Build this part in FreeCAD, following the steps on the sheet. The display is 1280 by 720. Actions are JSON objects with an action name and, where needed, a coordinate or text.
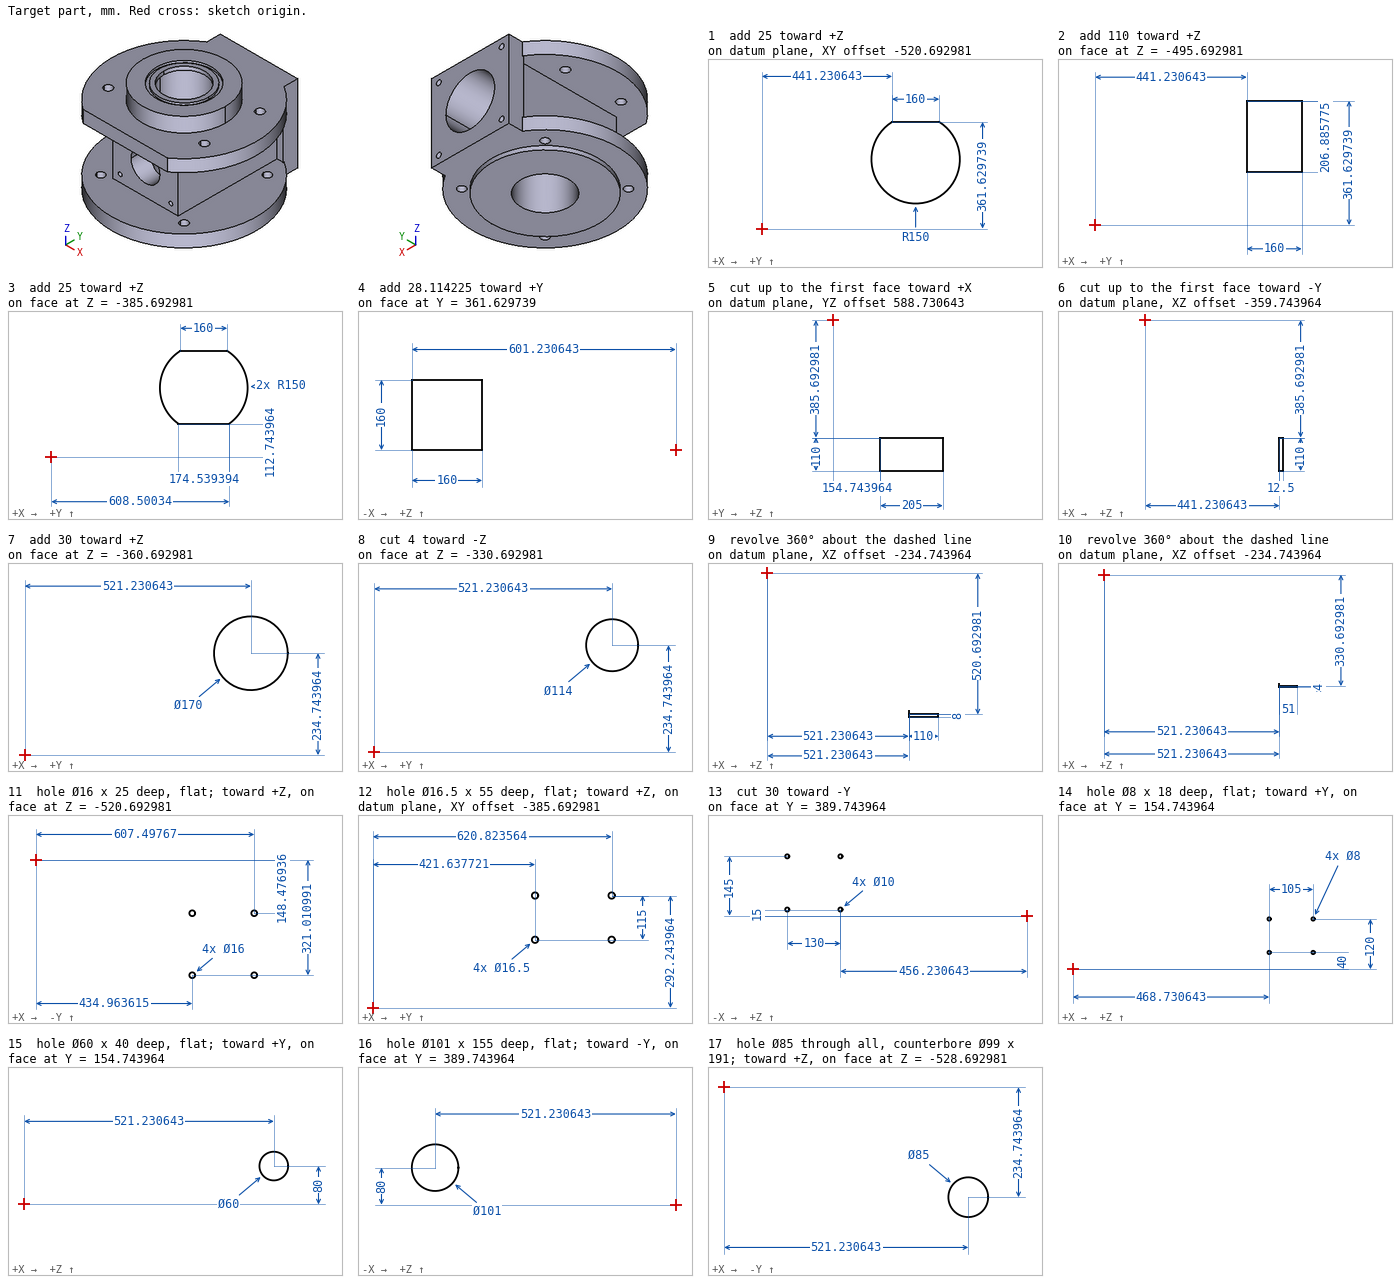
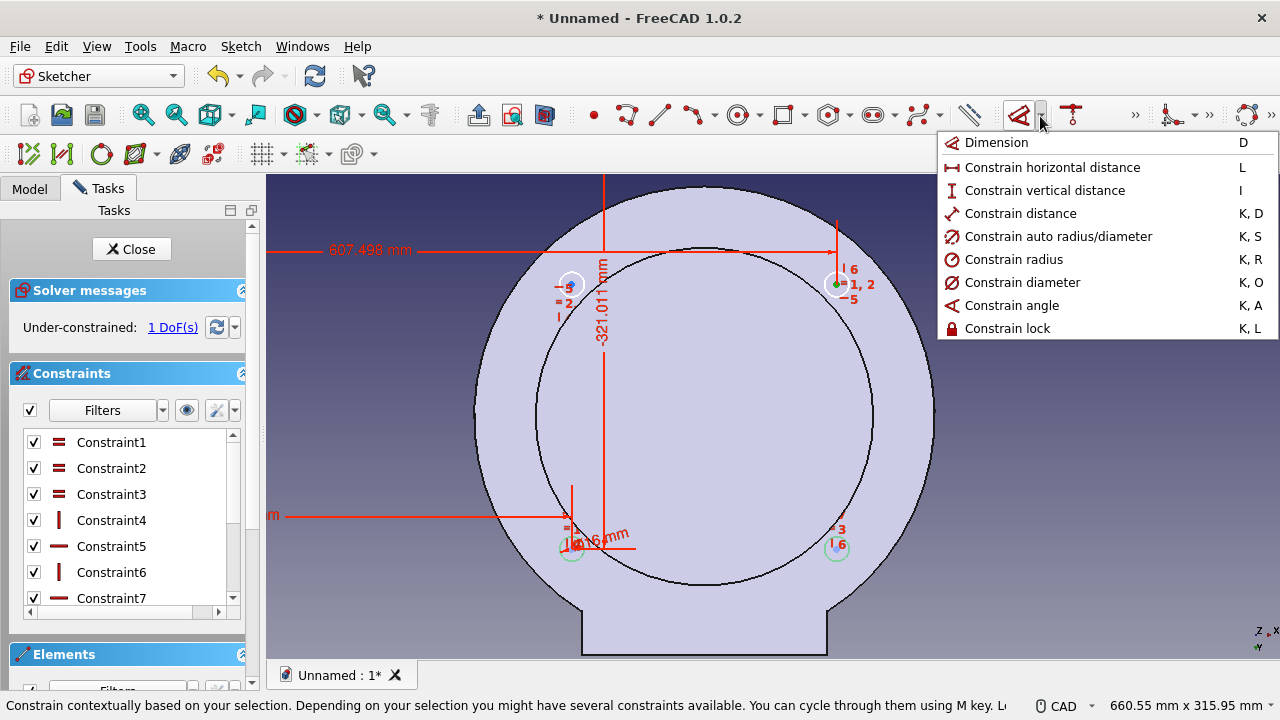
{"action": "left_click", "coordinate": [1108, 190]}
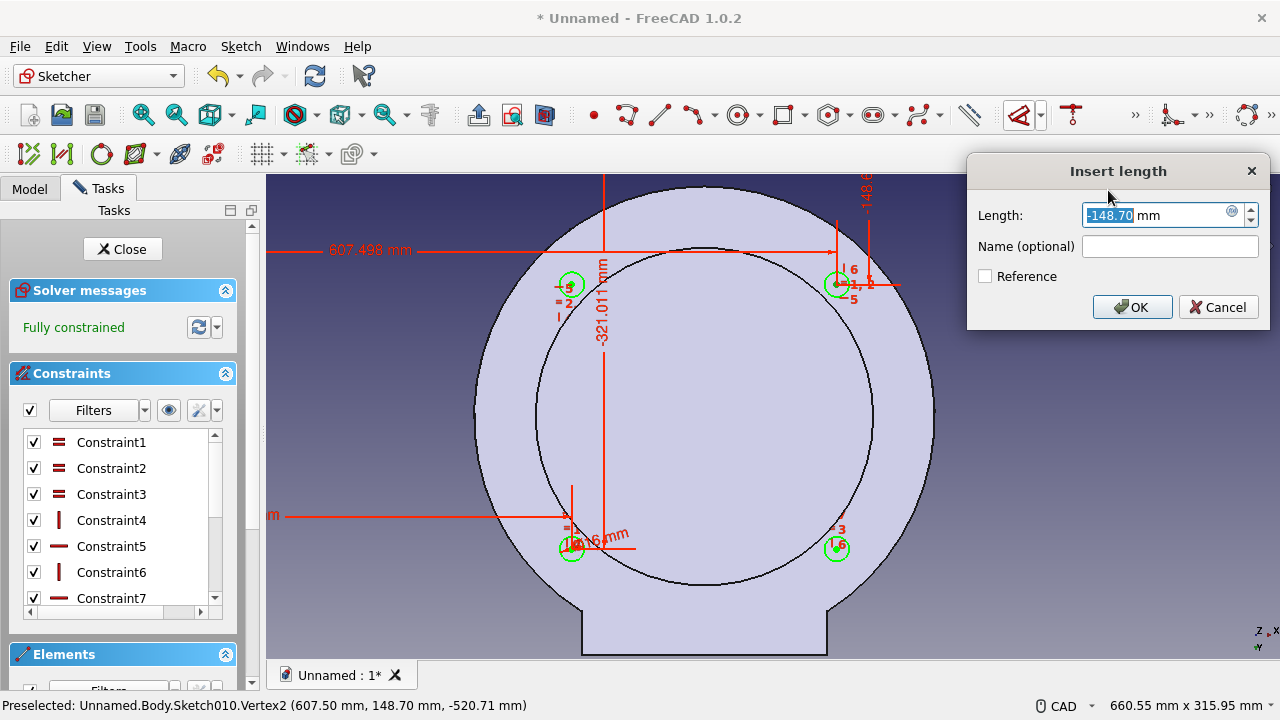
{"action": "type", "text": "-148.476936"}
{"action": "key", "text": "Return"}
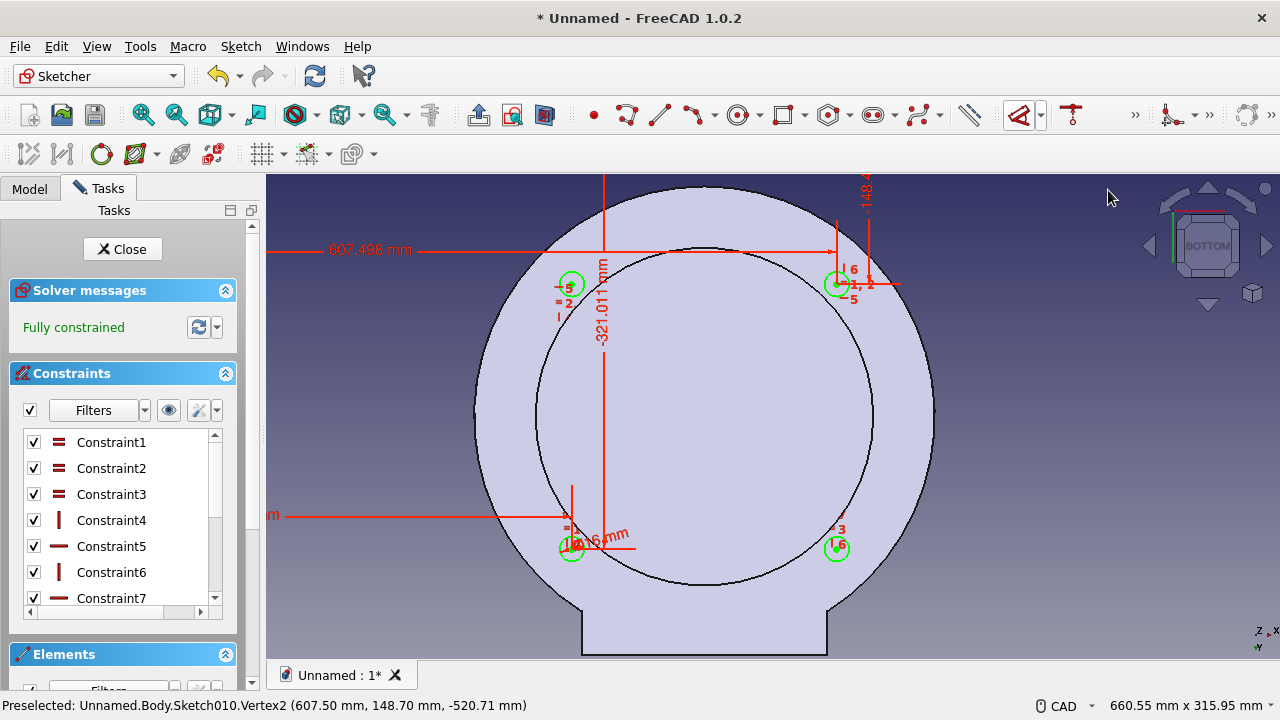
{"action": "left_click", "coordinate": [123, 249]}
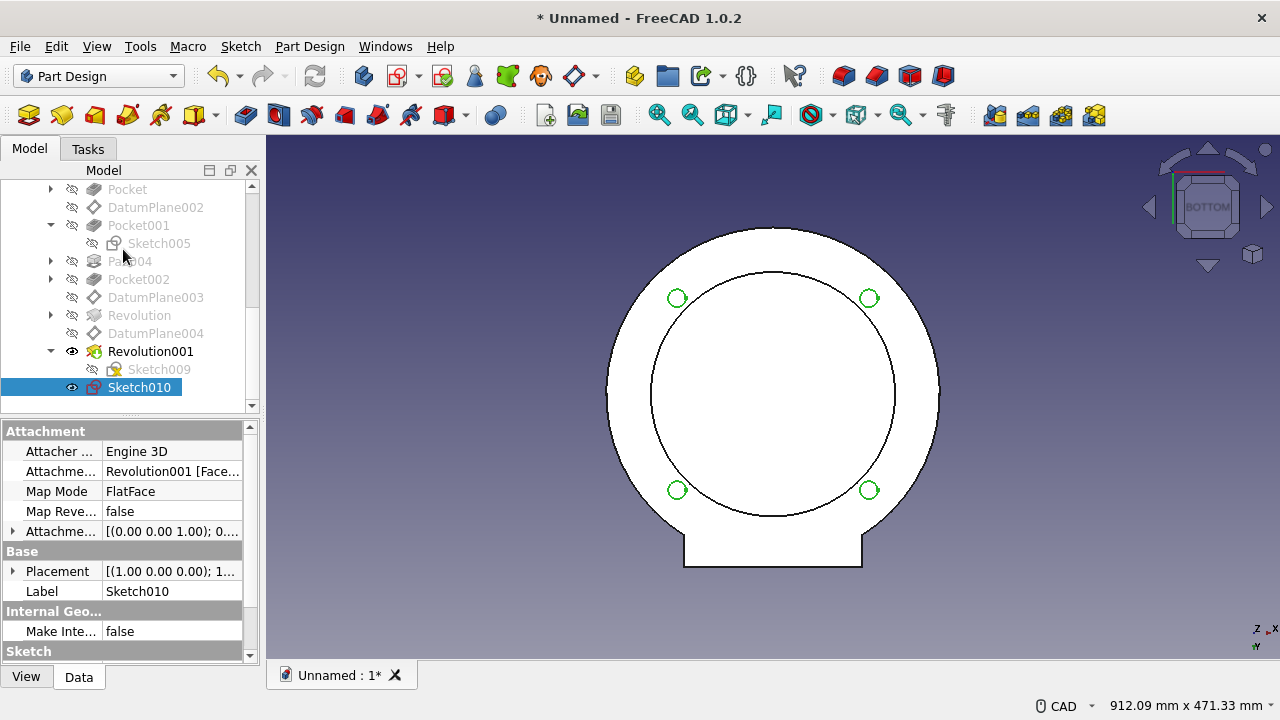
{"action": "left_click", "coordinate": [279, 116]}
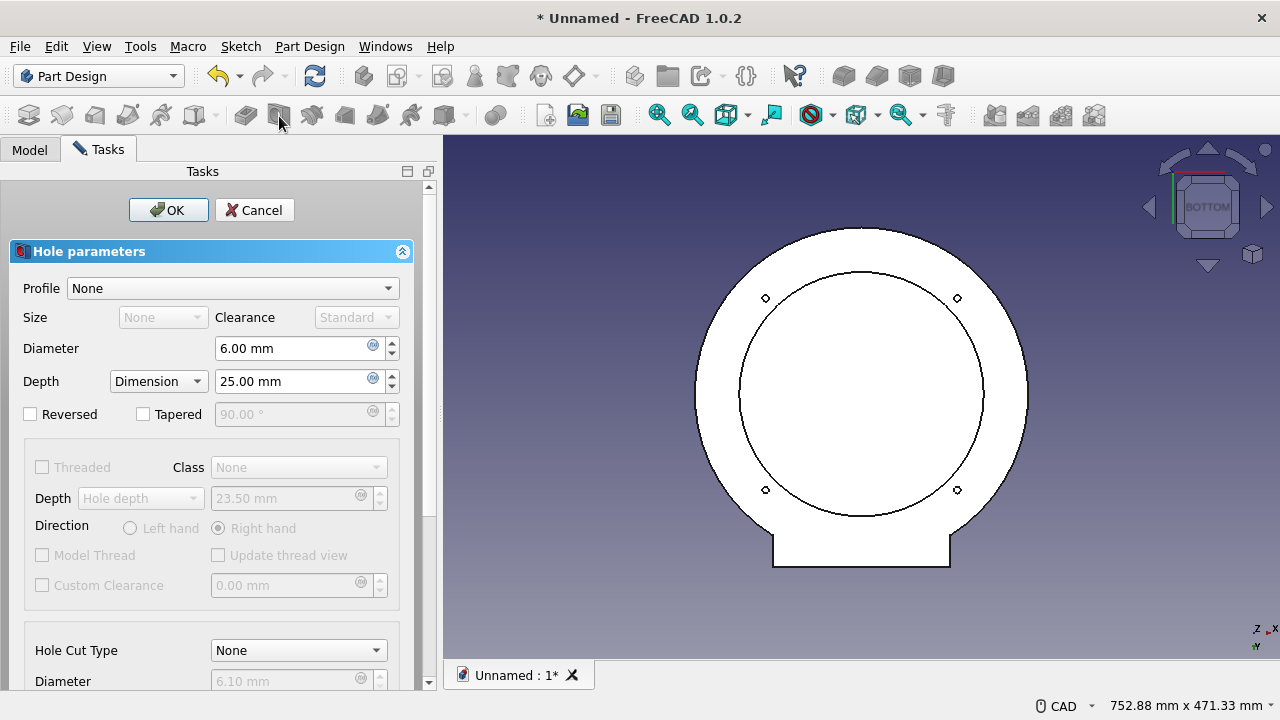
{"action": "triple_click", "coordinate": [300, 348]}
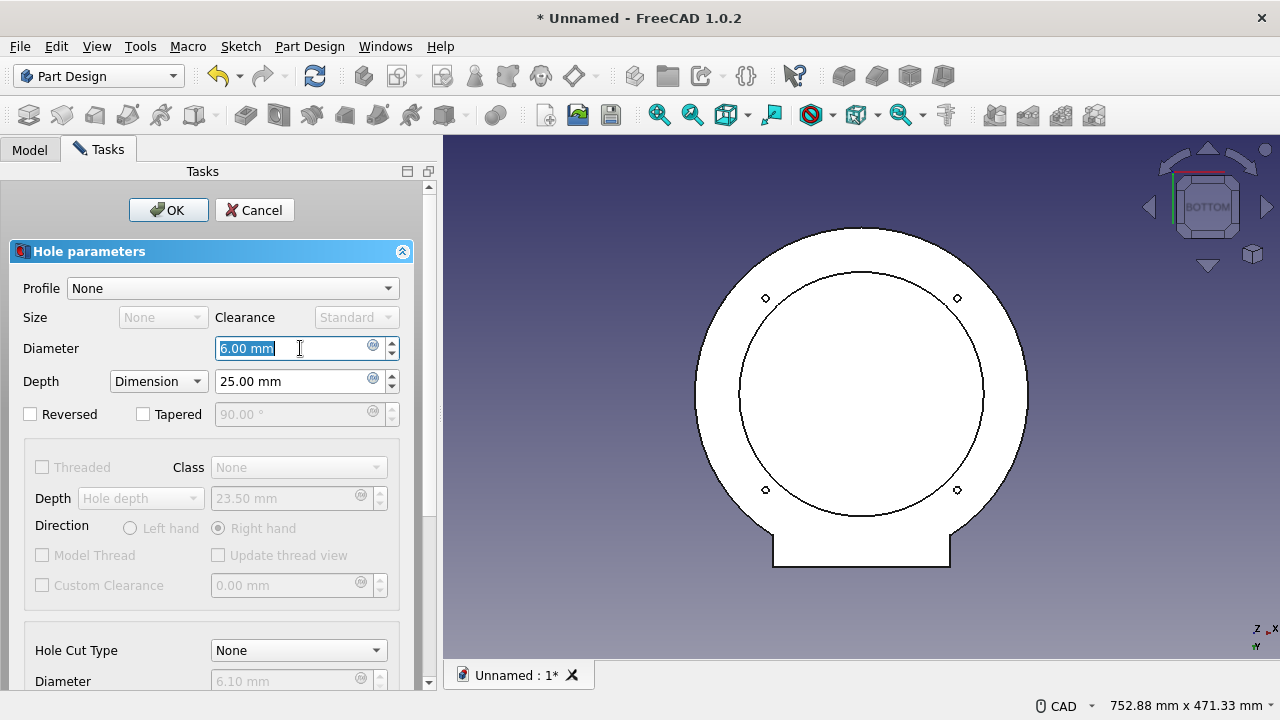
{"action": "type", "text": "16"}
{"action": "key", "text": "Tab"}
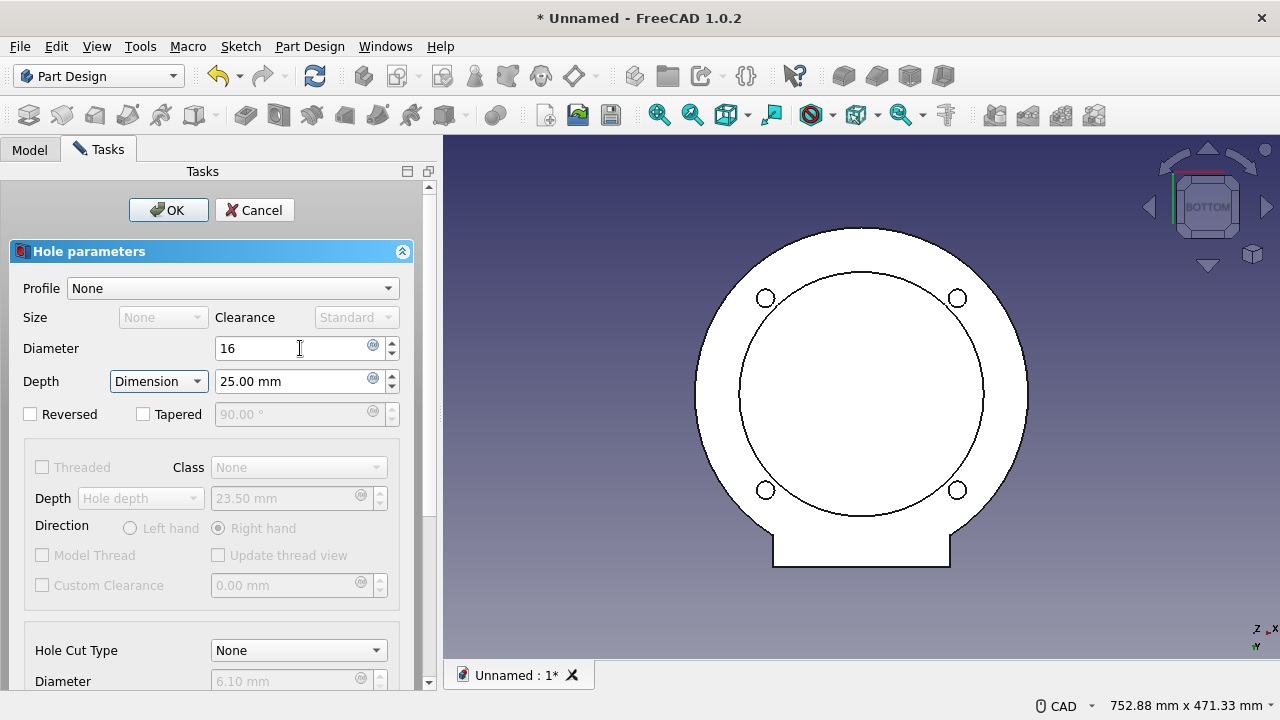
{"action": "triple_click", "coordinate": [300, 382]}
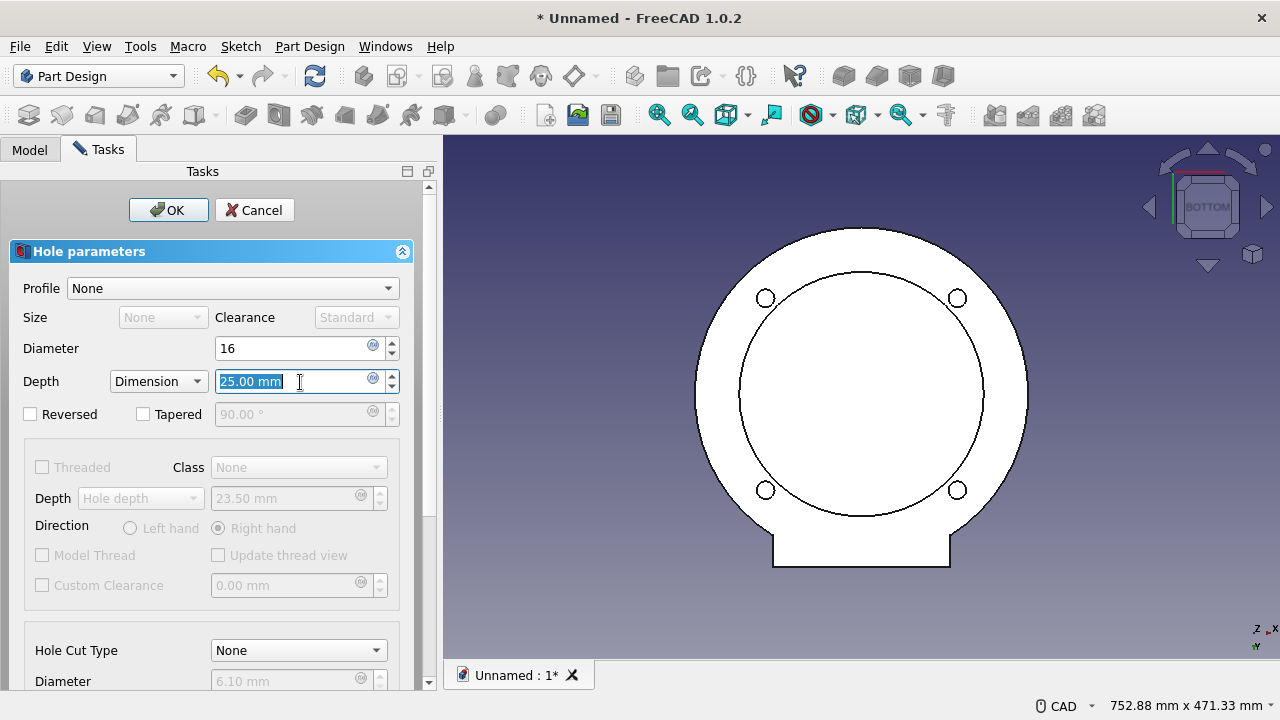
{"action": "type", "text": "25"}
{"action": "key", "text": "Tab"}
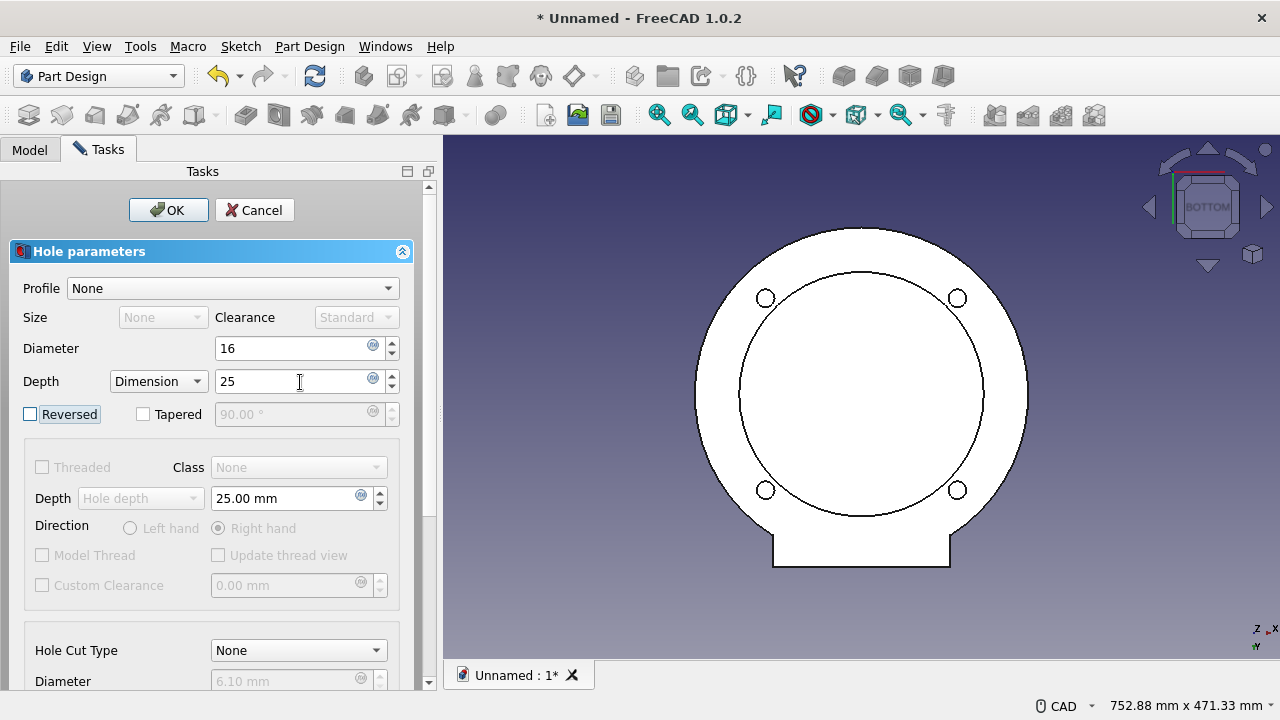
{"action": "scroll", "coordinate": [429, 436], "scroll_direction": "down", "scroll_amount": 4}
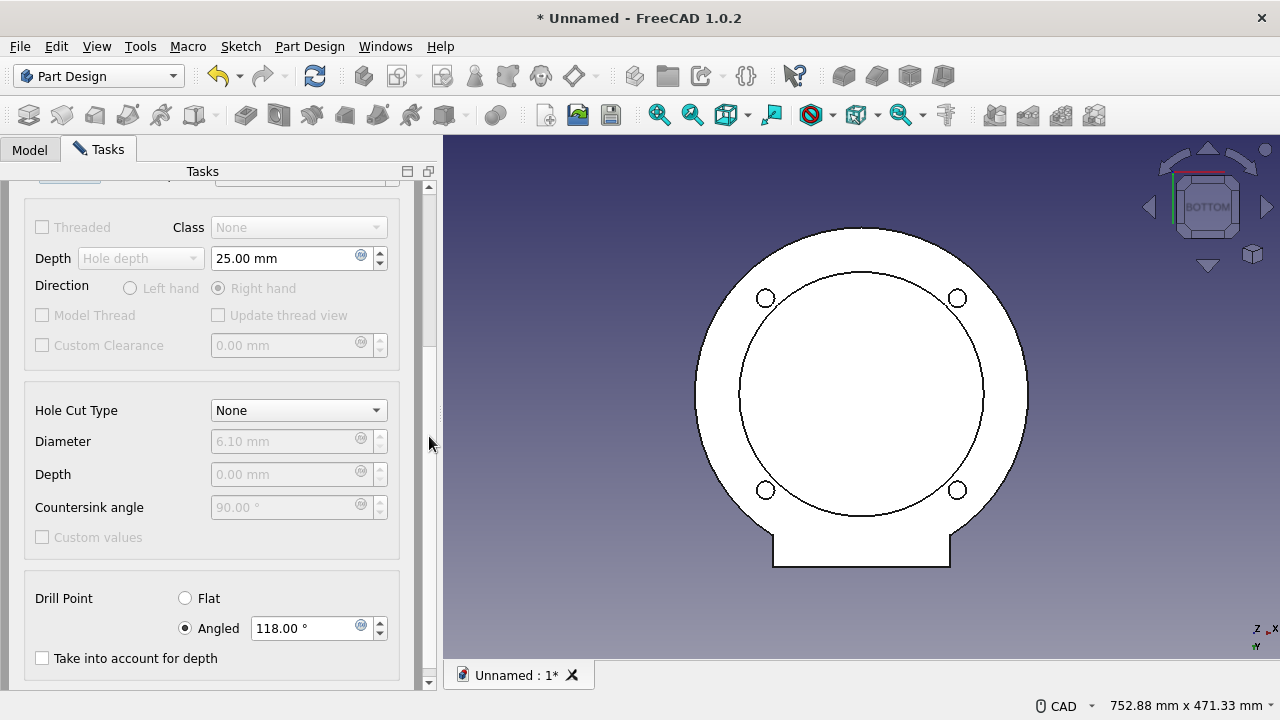
{"action": "left_click", "coordinate": [186, 596]}